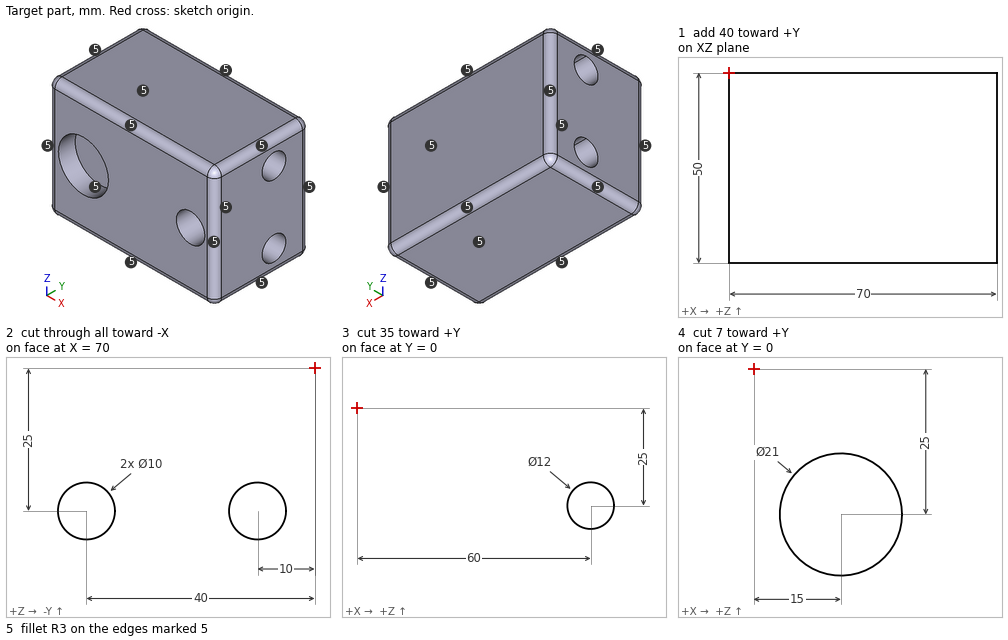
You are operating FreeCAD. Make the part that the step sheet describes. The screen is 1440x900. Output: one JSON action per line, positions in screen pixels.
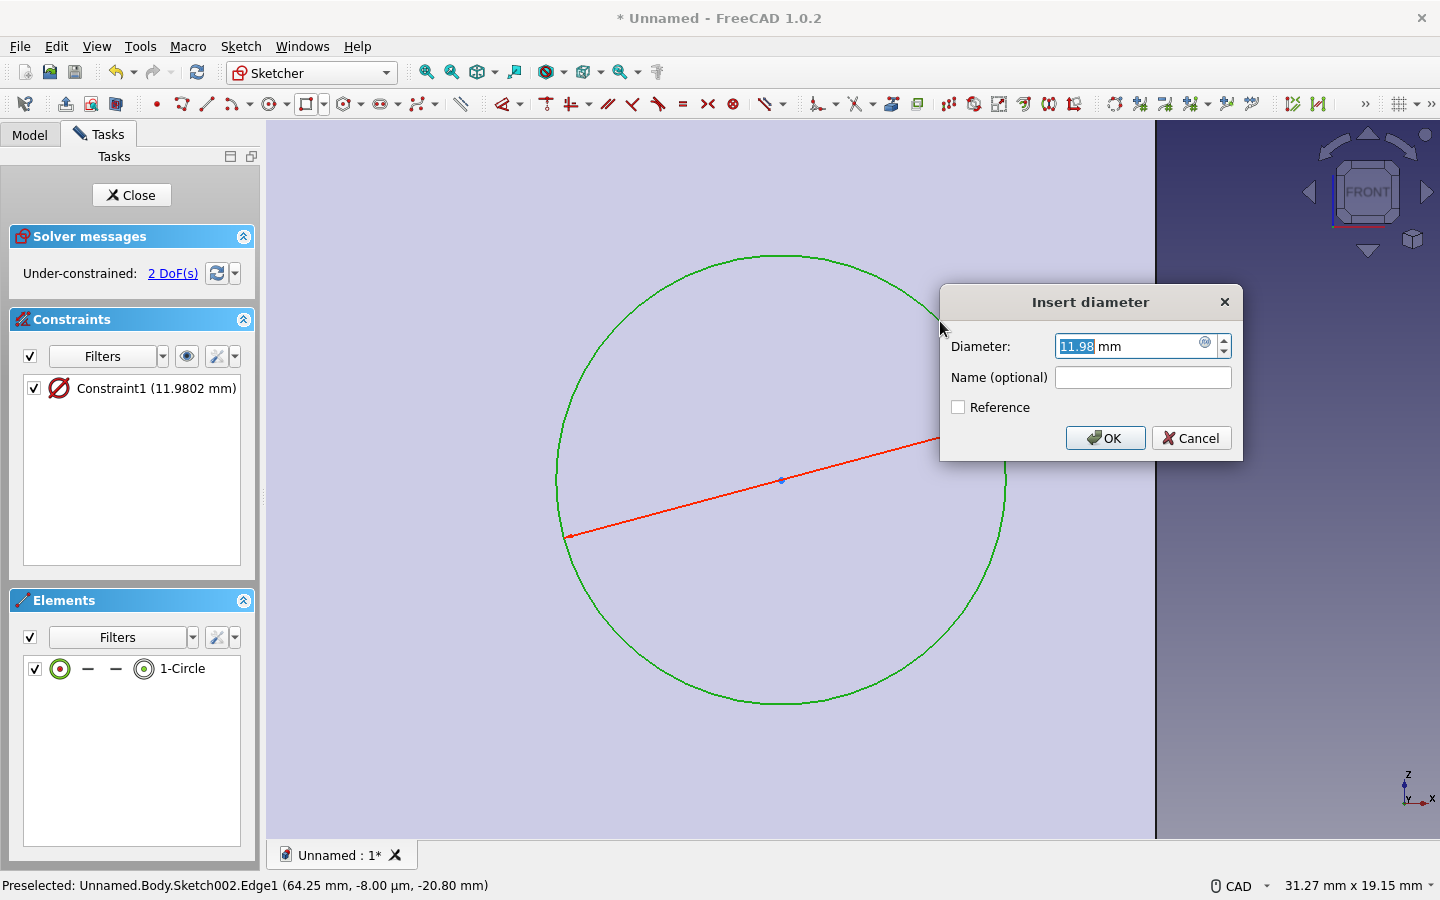
{"action": "type", "text": "12"}
{"action": "key", "text": "Return"}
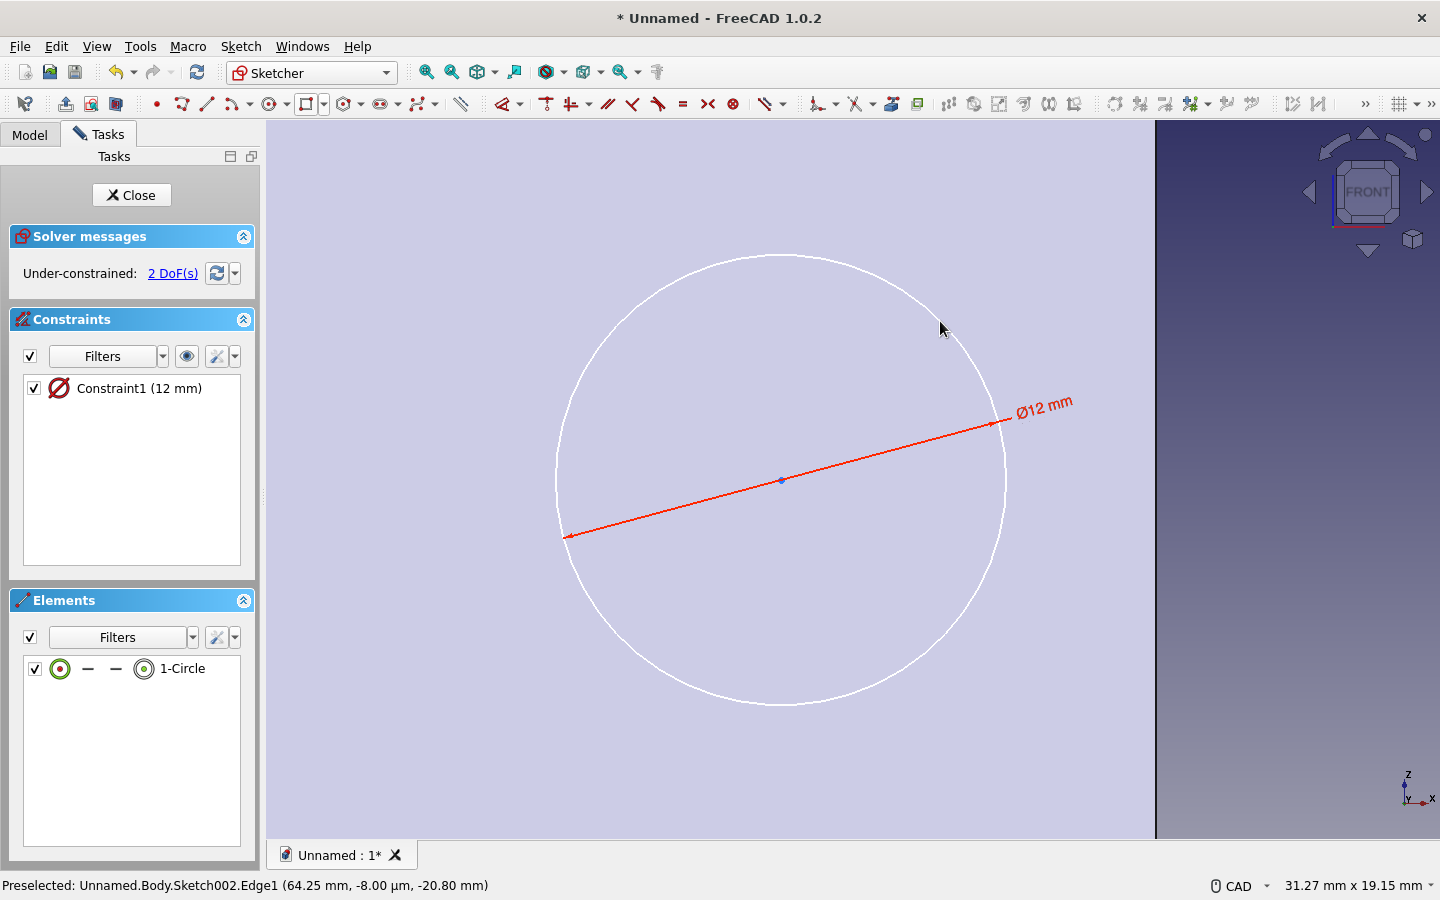
{"action": "left_click", "coordinate": [781, 480]}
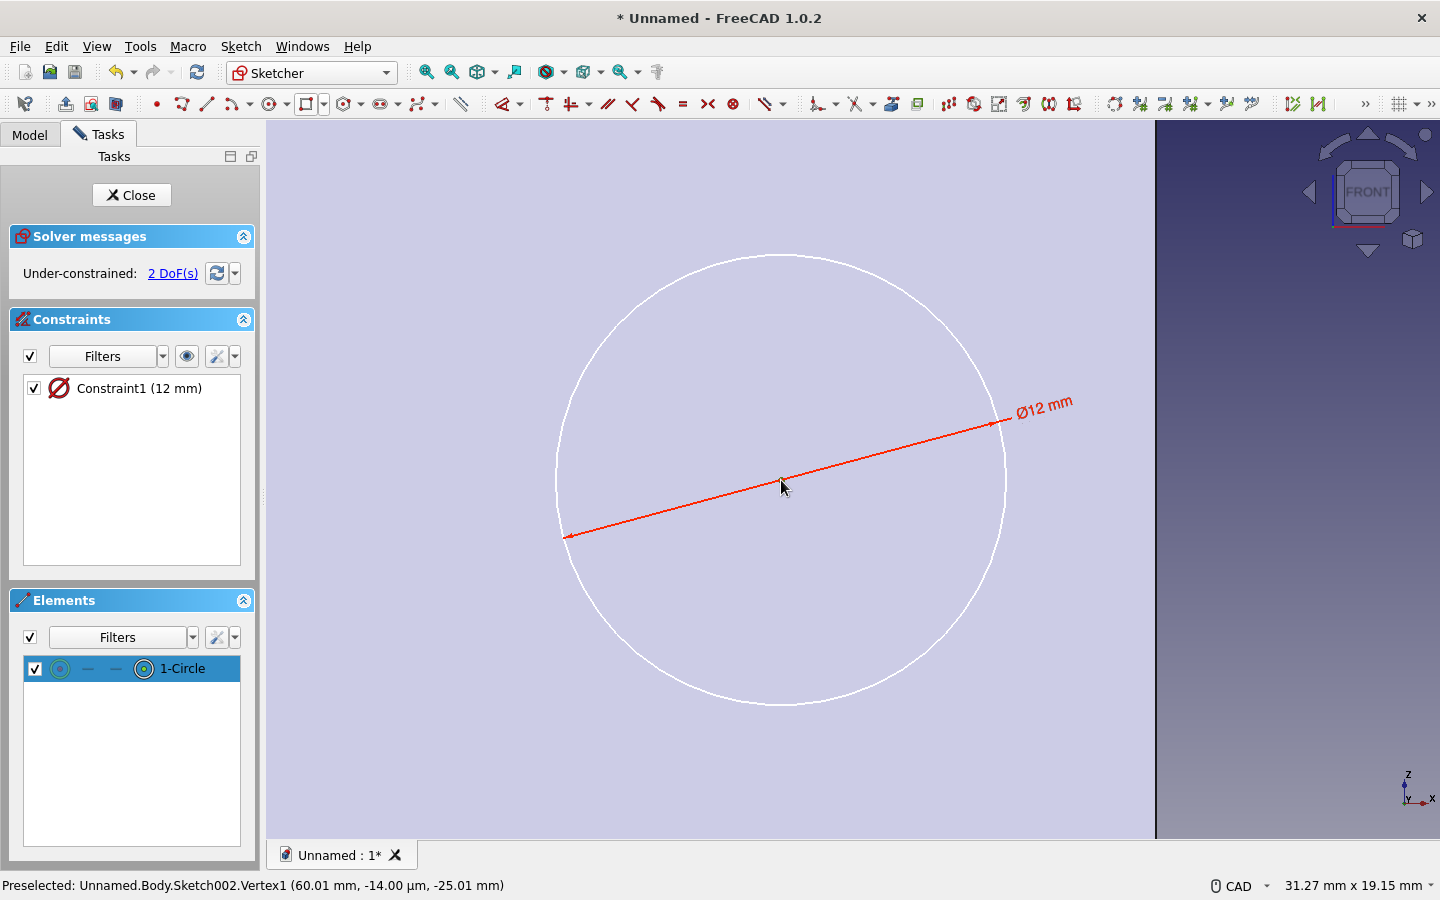
{"action": "key", "text": "l"}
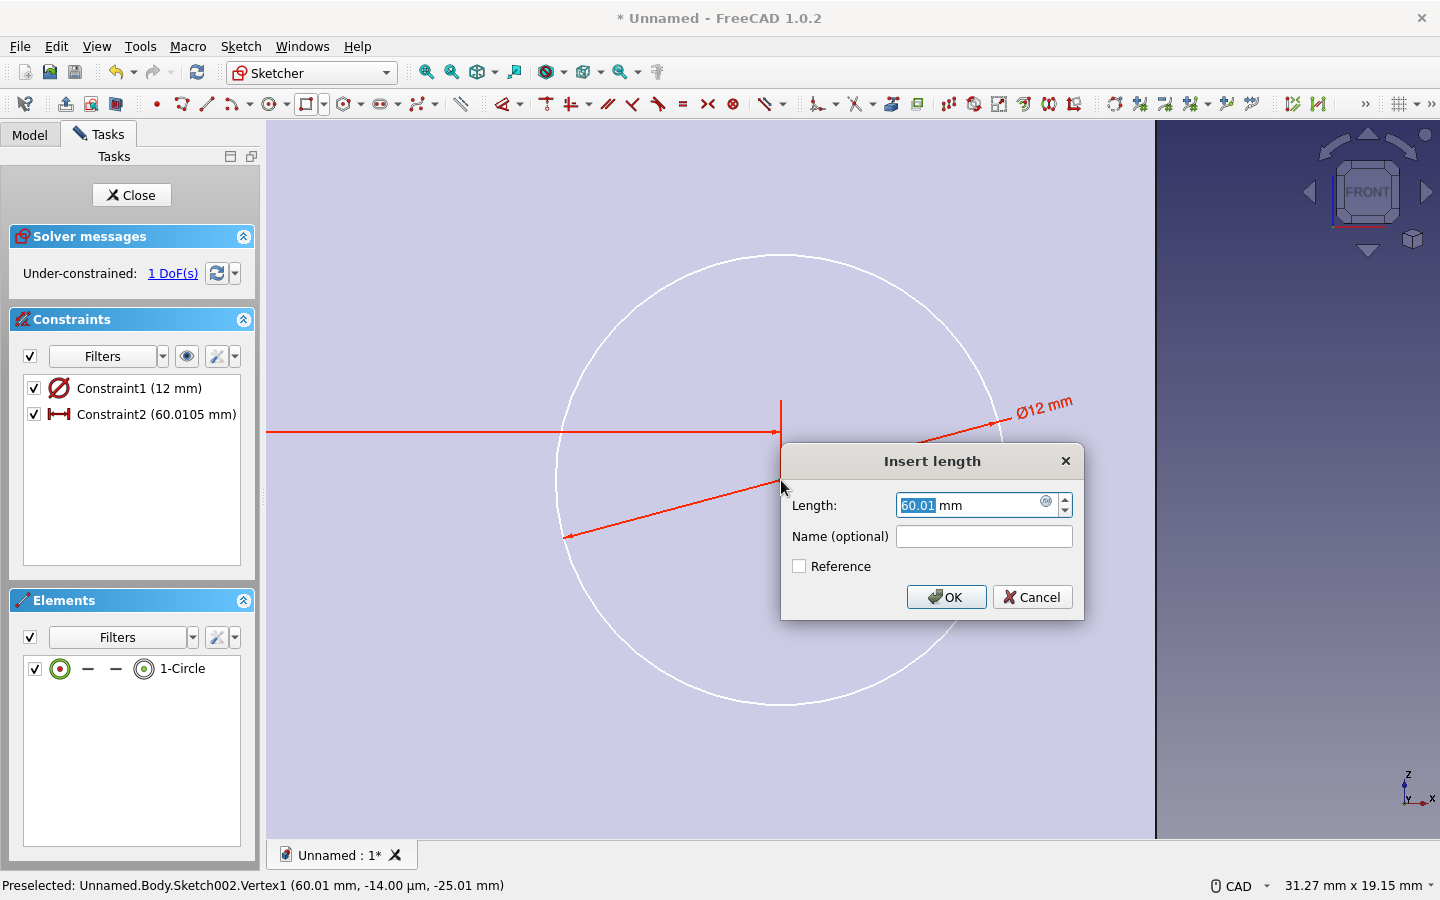
{"action": "type", "text": "60"}
{"action": "key", "text": "Return"}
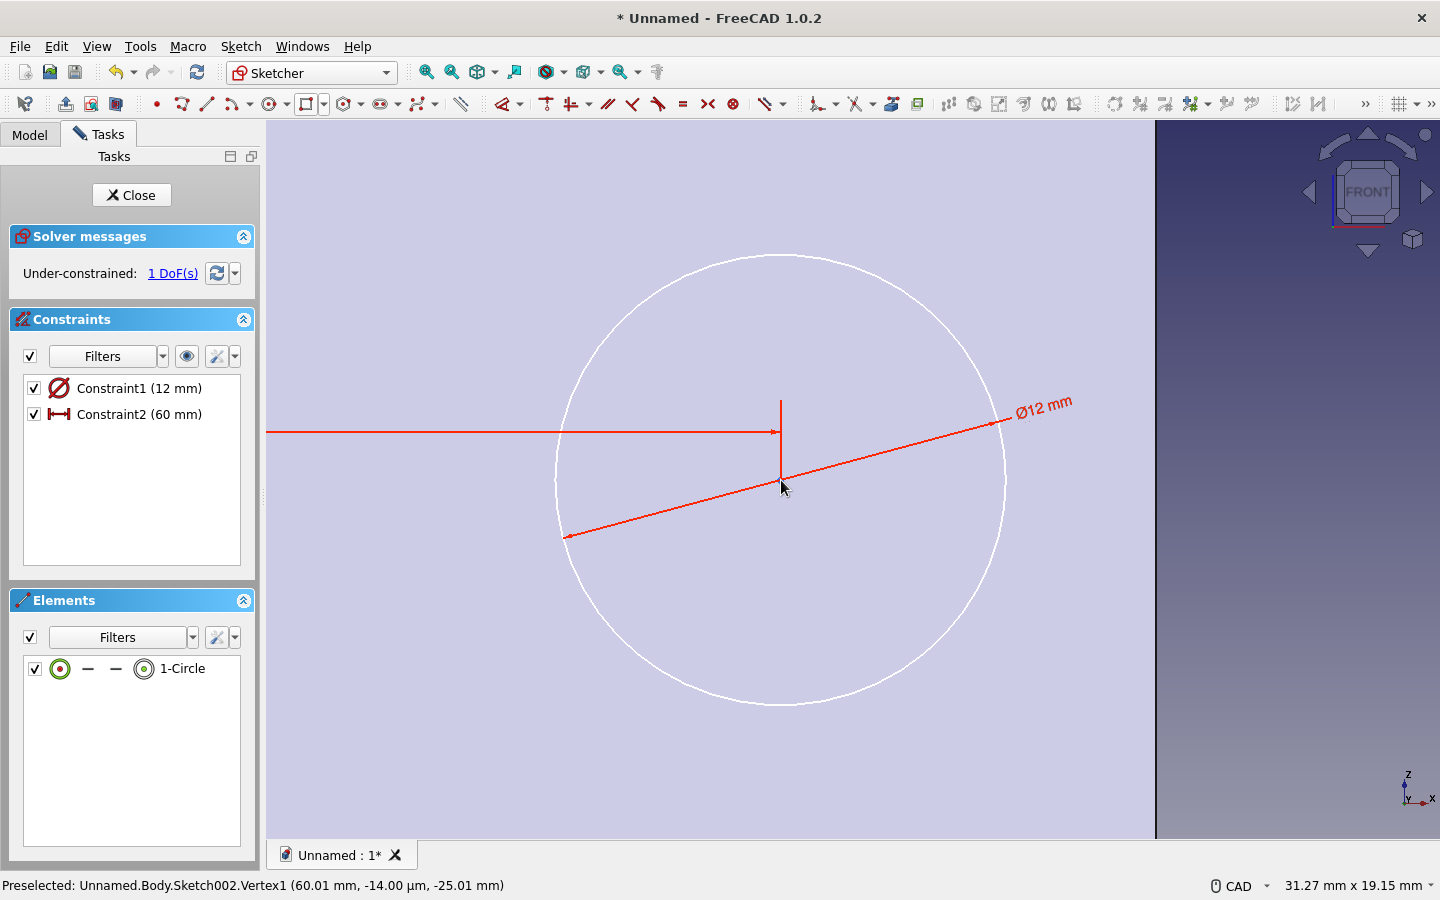
{"action": "left_click", "coordinate": [781, 480]}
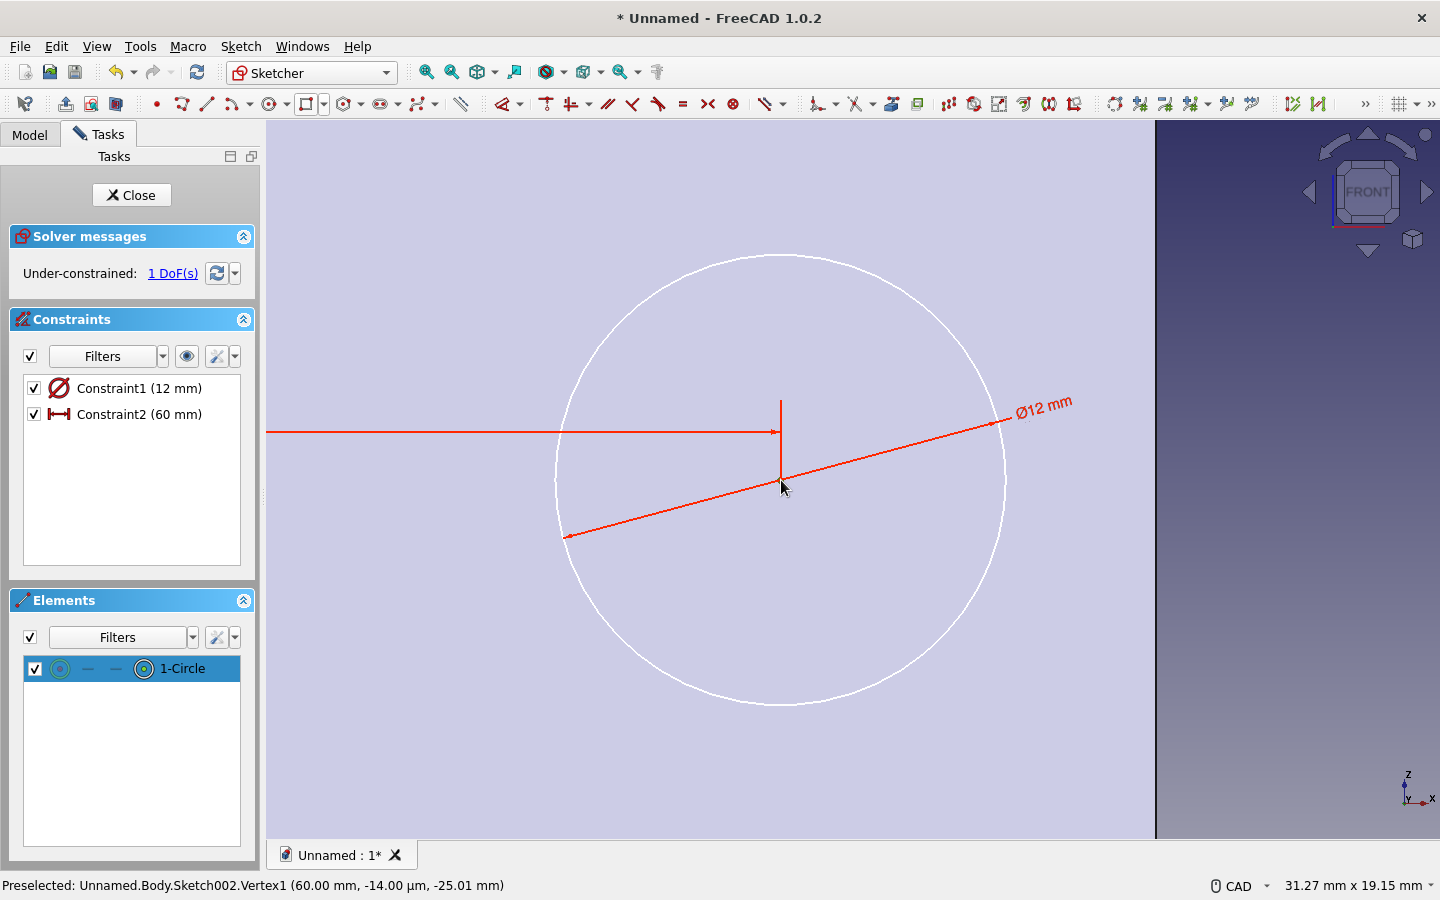
{"action": "key", "text": "i"}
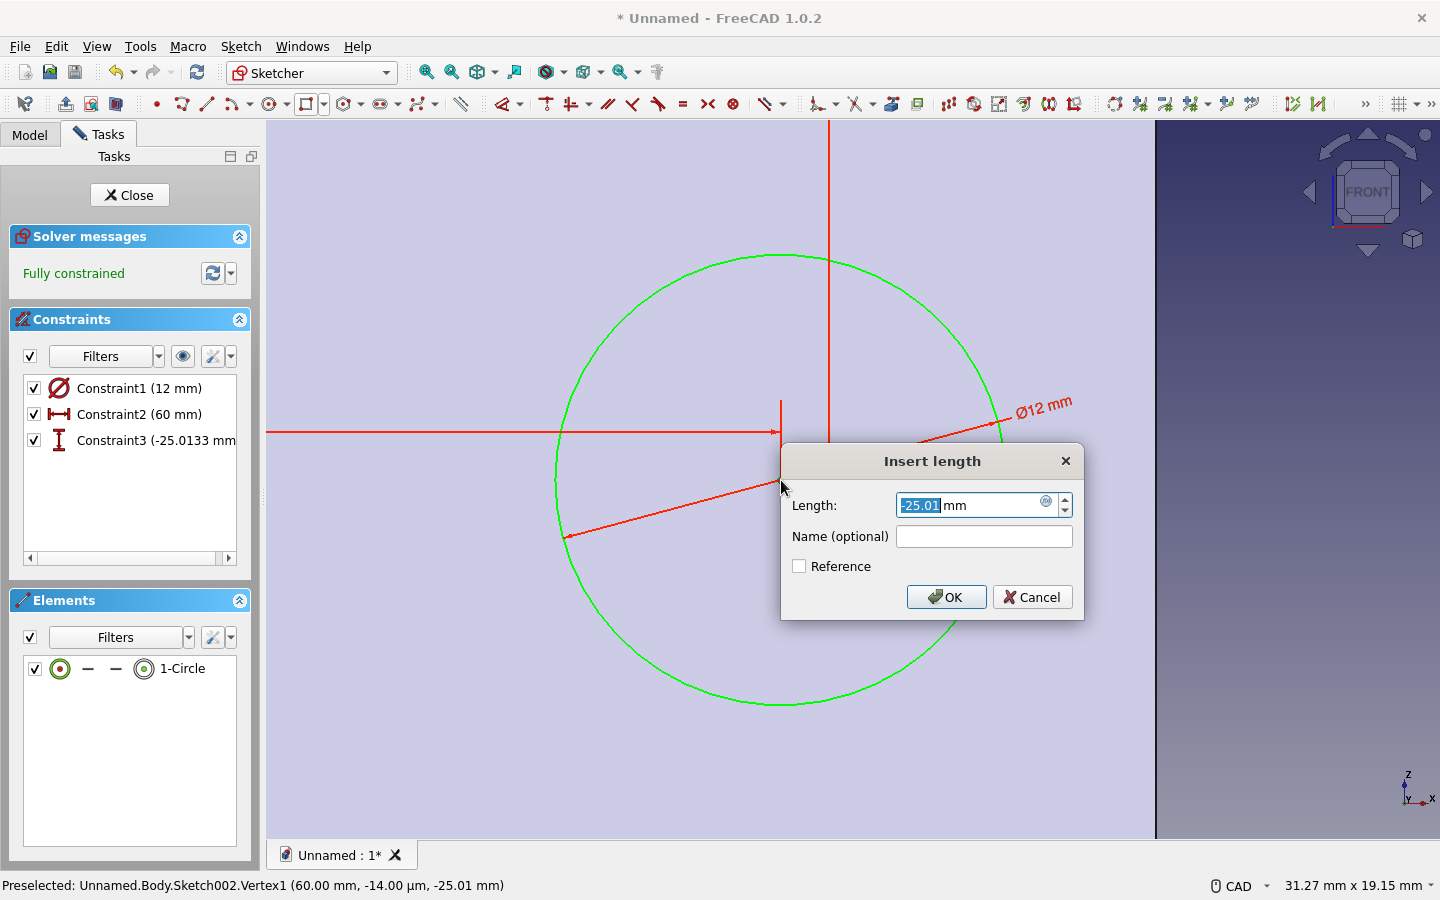
{"action": "type", "text": "-25"}
{"action": "key", "text": "Return"}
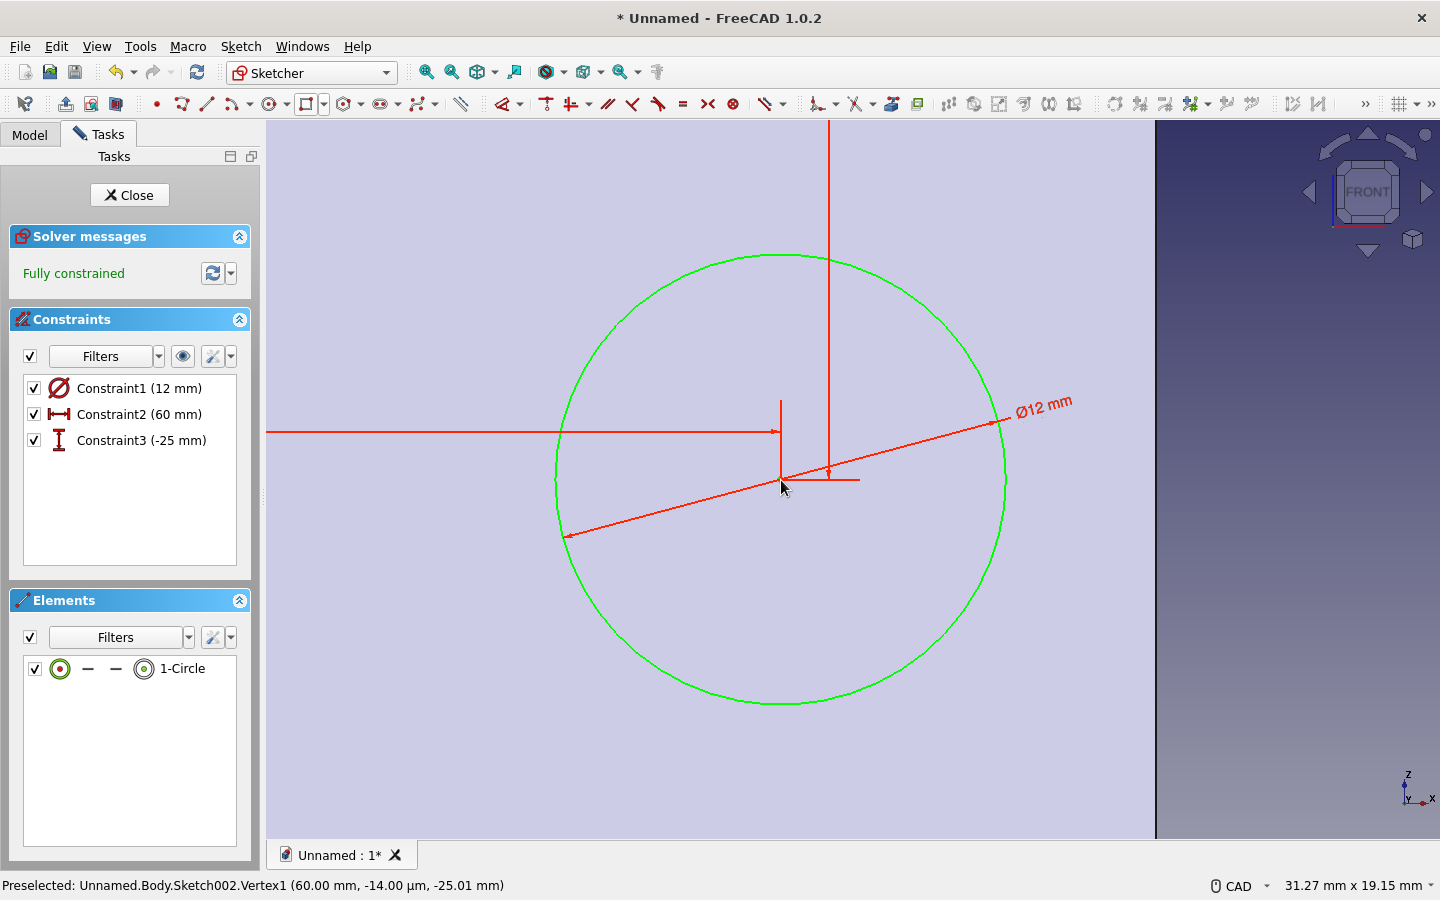
{"action": "left_click", "coordinate": [130, 195]}